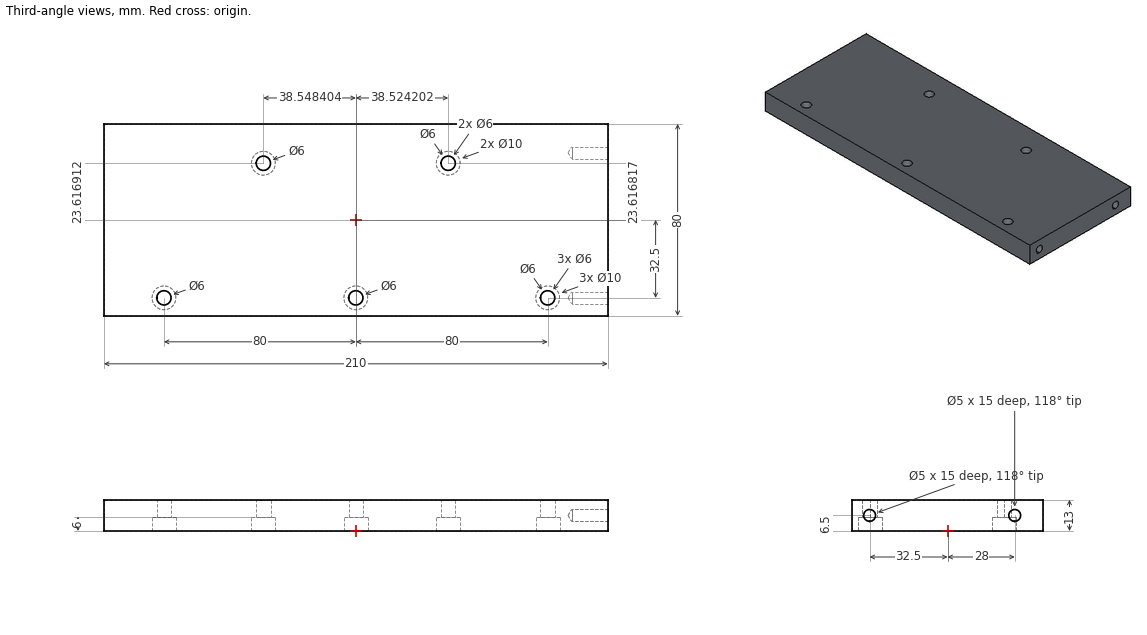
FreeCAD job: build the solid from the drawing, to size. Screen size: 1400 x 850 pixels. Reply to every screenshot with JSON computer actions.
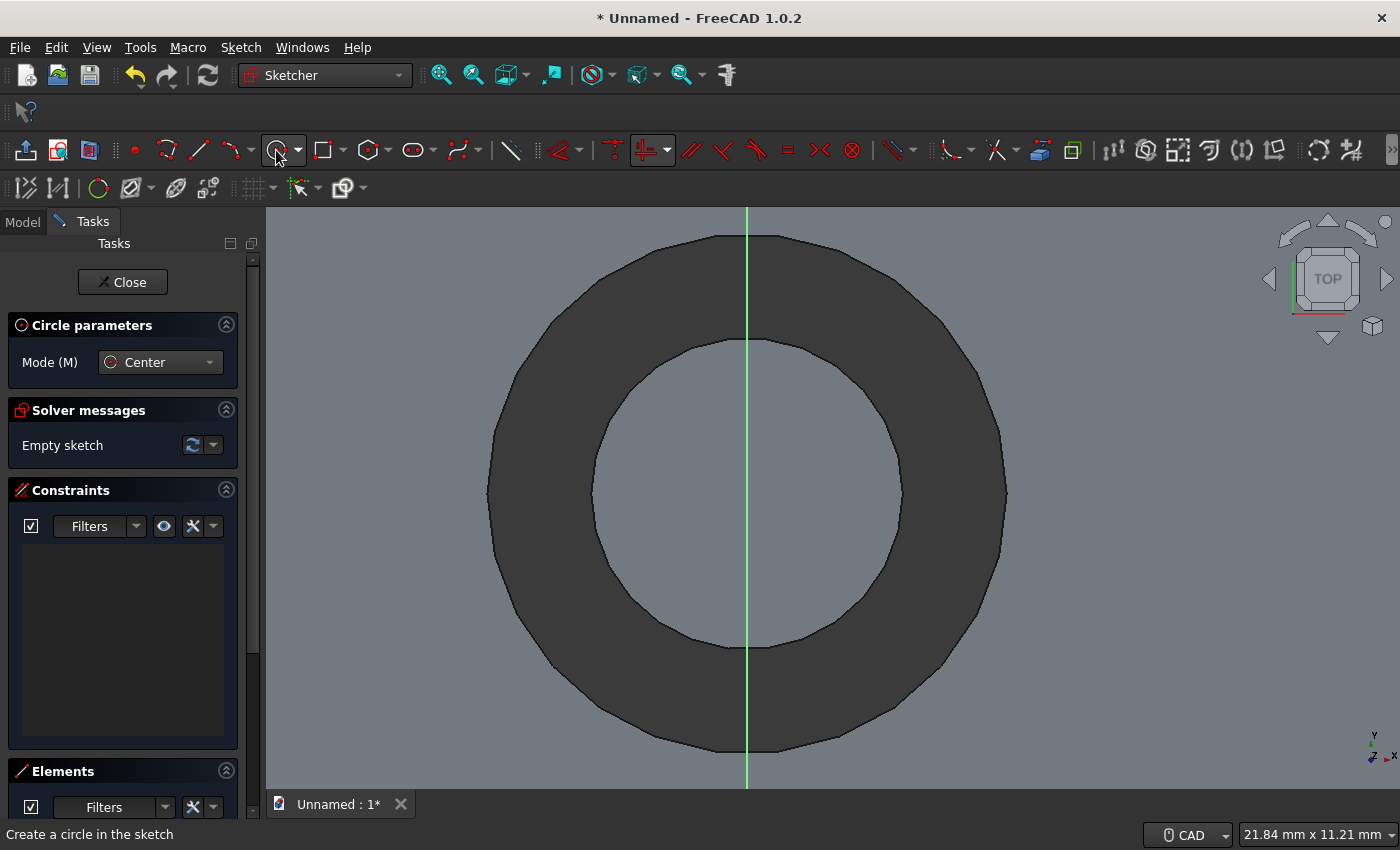
{"action": "left_click", "coordinate": [747, 494]}
{"action": "left_click", "coordinate": [857, 384]}
{"action": "key", "text": "Escape"}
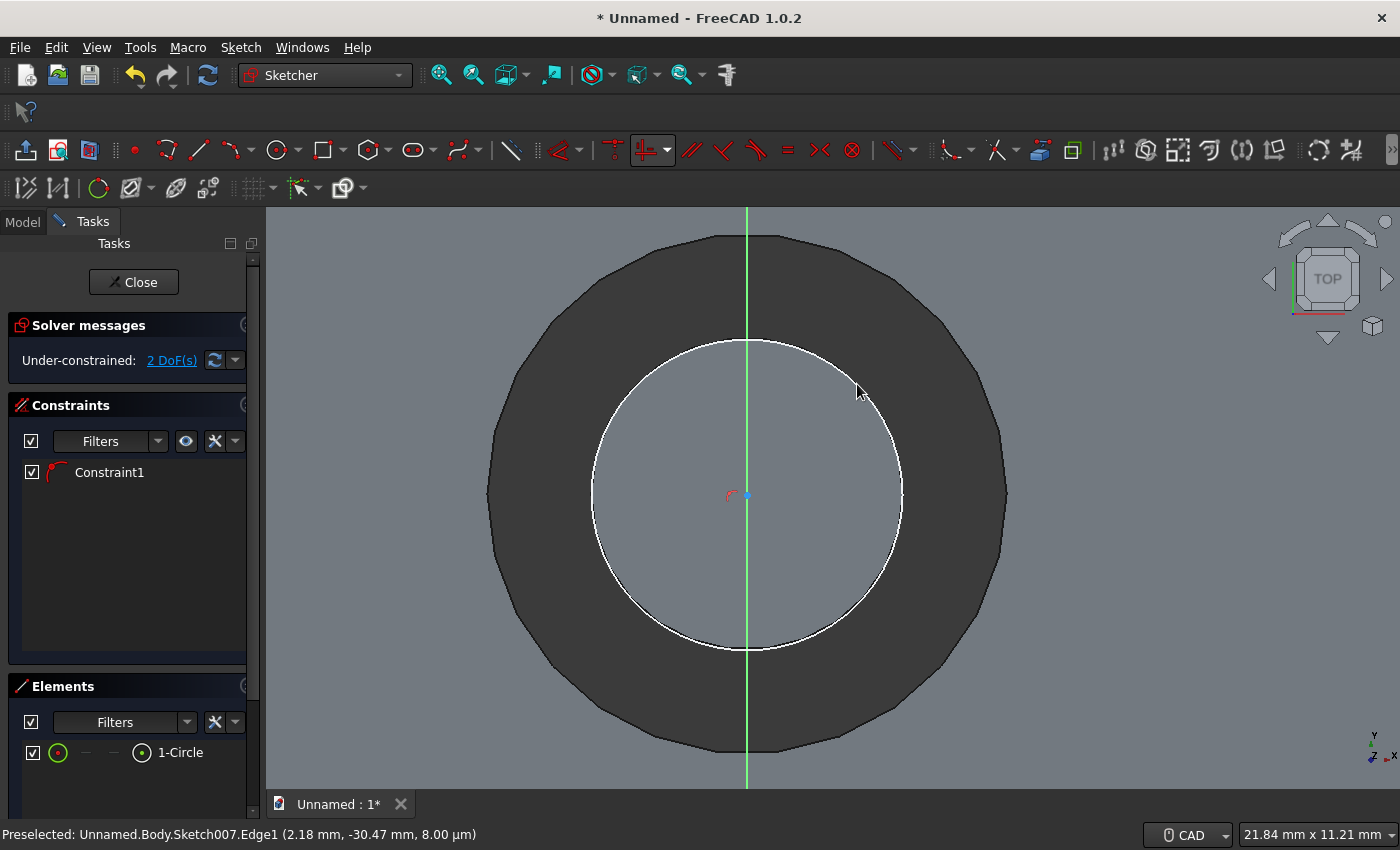
{"action": "key", "text": "d"}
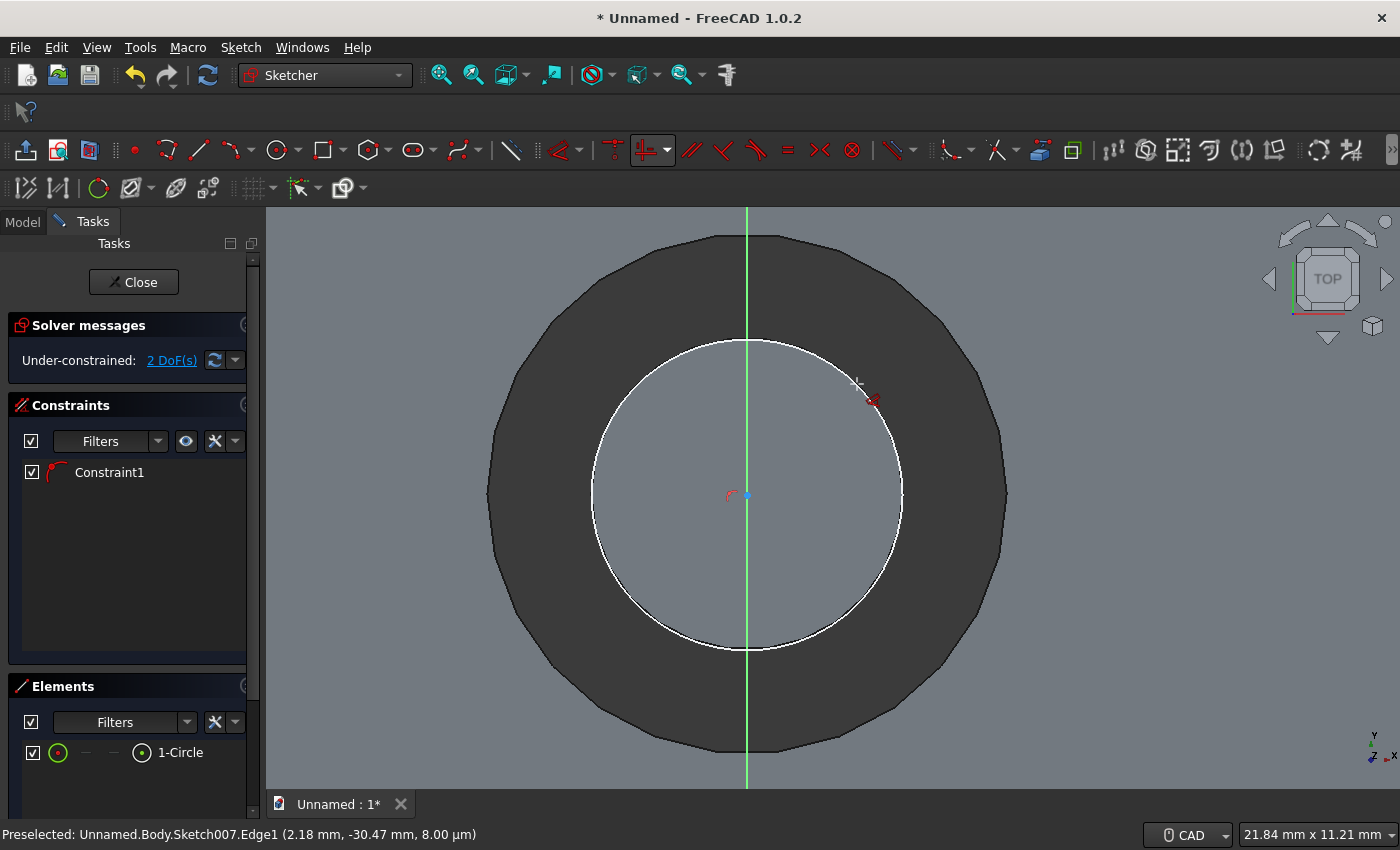
{"action": "left_click", "coordinate": [857, 385]}
{"action": "left_click", "coordinate": [880, 362]}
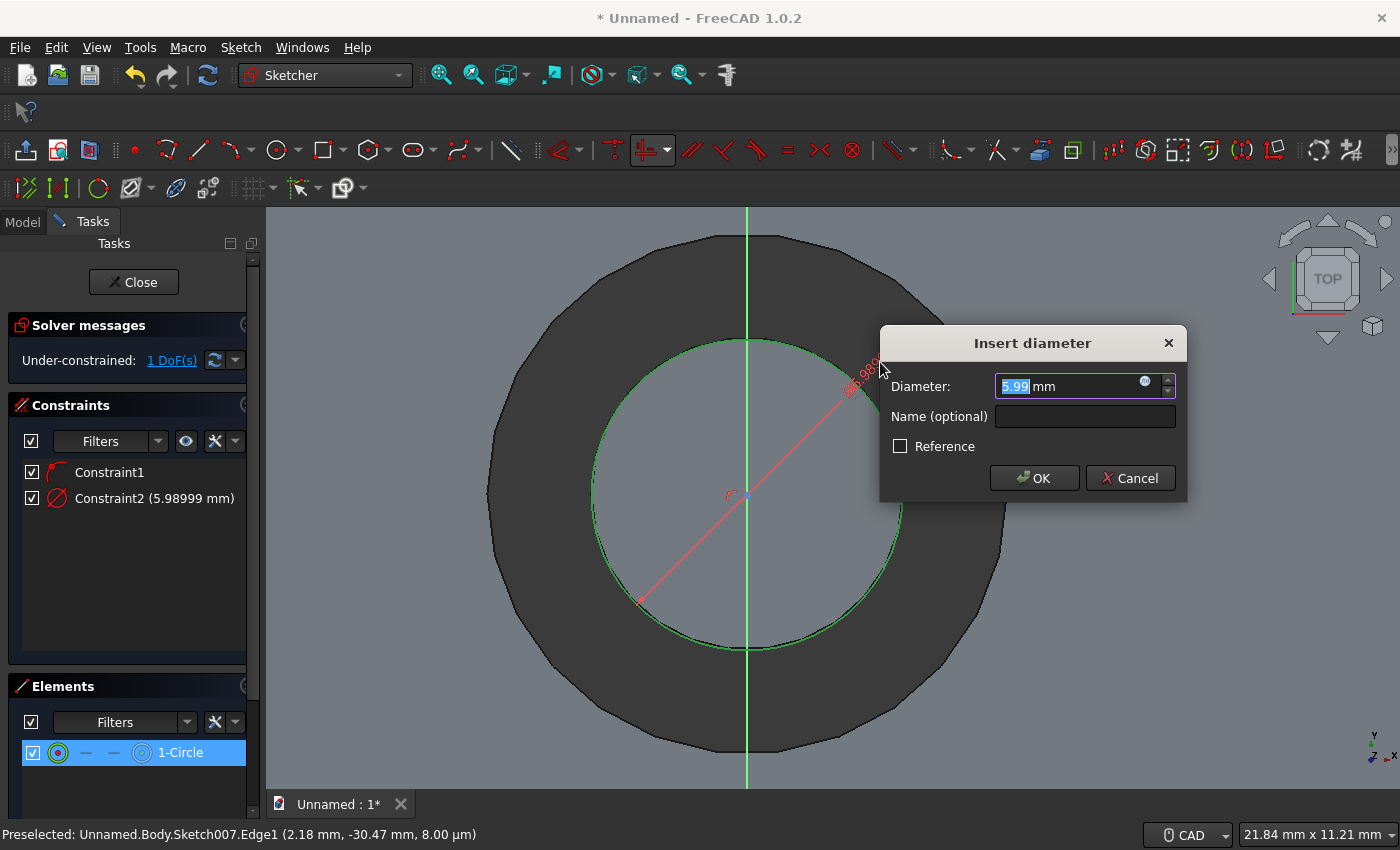
{"action": "type", "text": "6"}
{"action": "key", "text": "Return"}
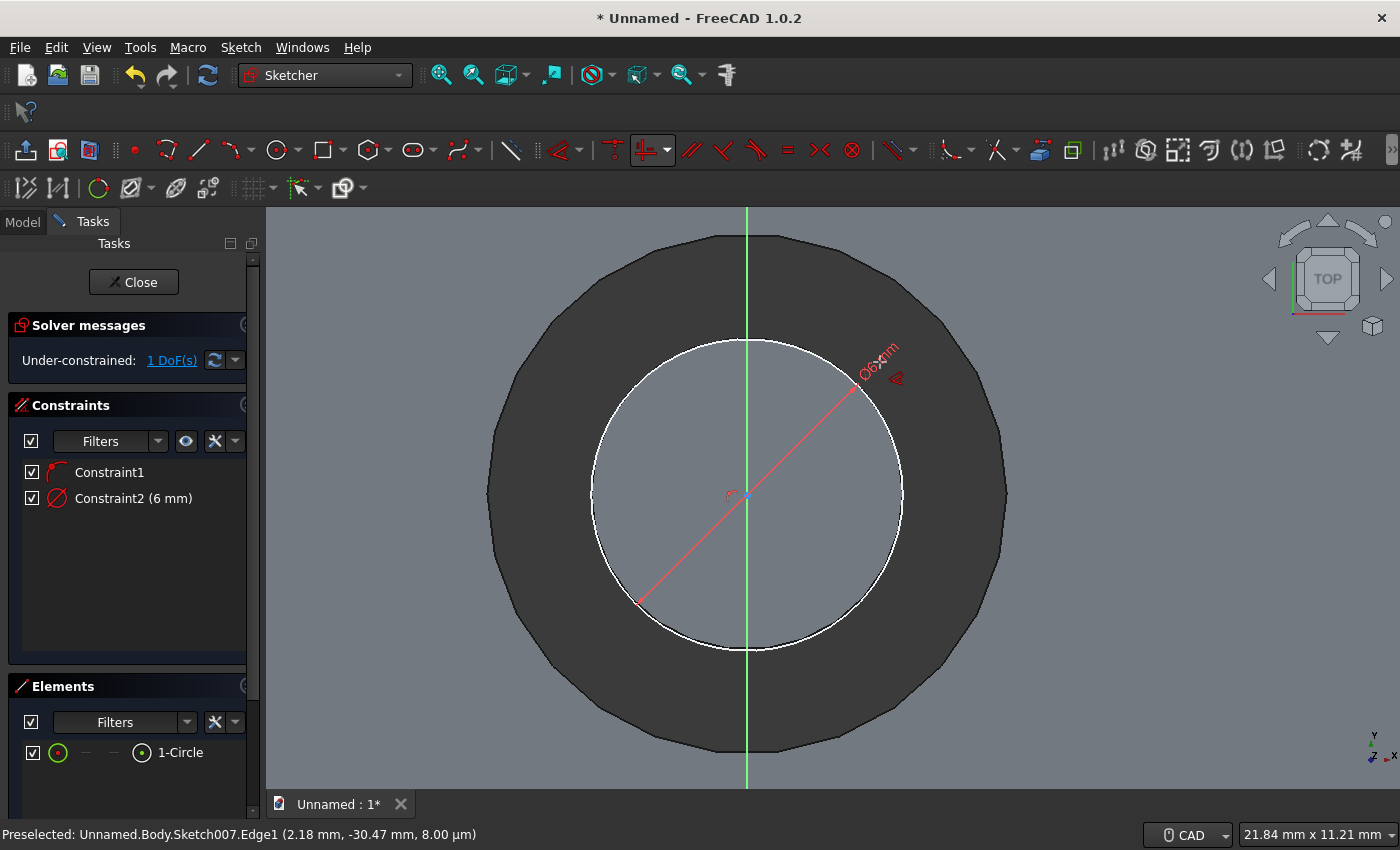
{"action": "left_click", "coordinate": [747, 495]}
{"action": "left_click", "coordinate": [781, 365]}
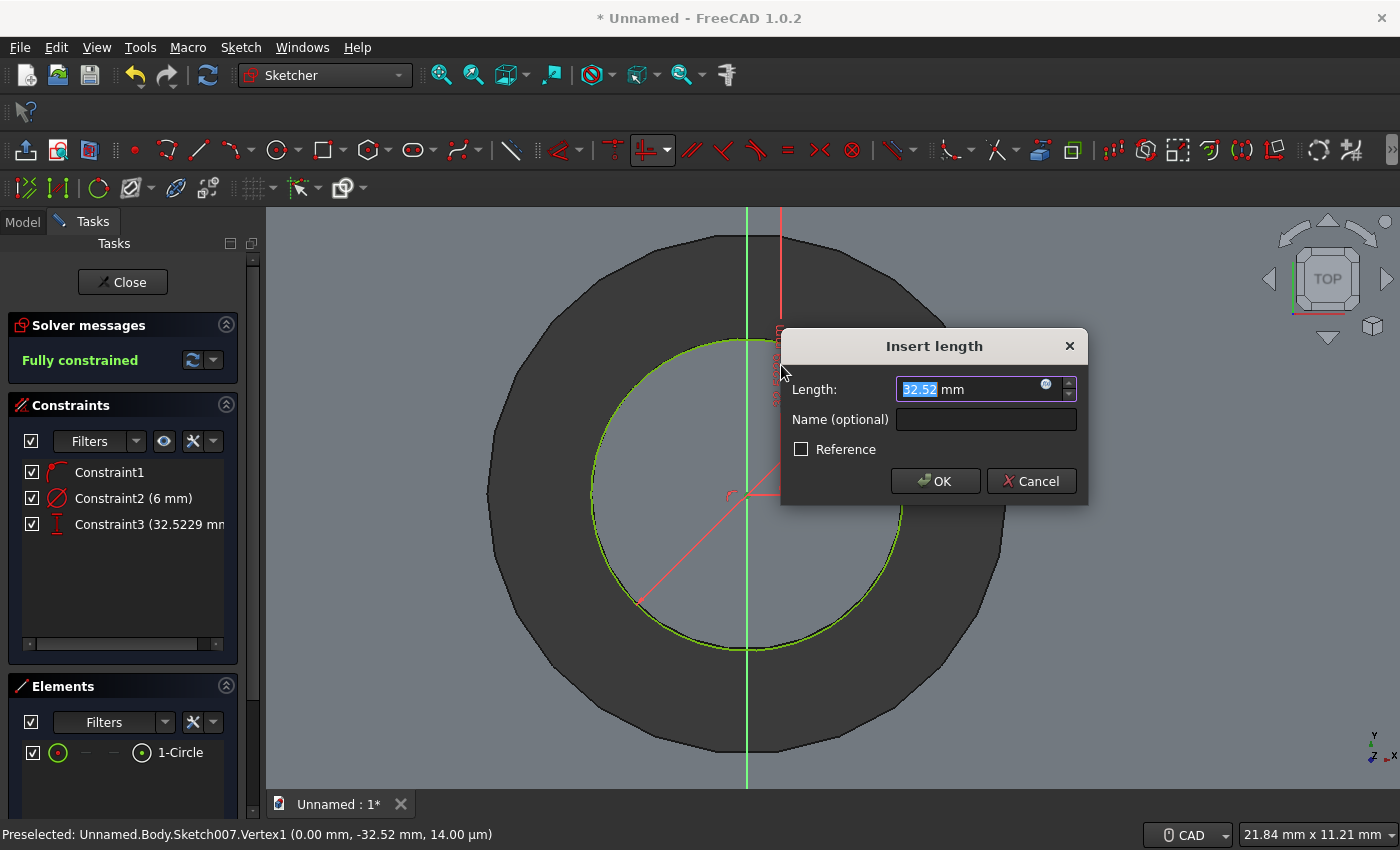
{"action": "type", "text": "32.5"}
{"action": "key", "text": "Return"}
{"action": "key", "text": "Escape"}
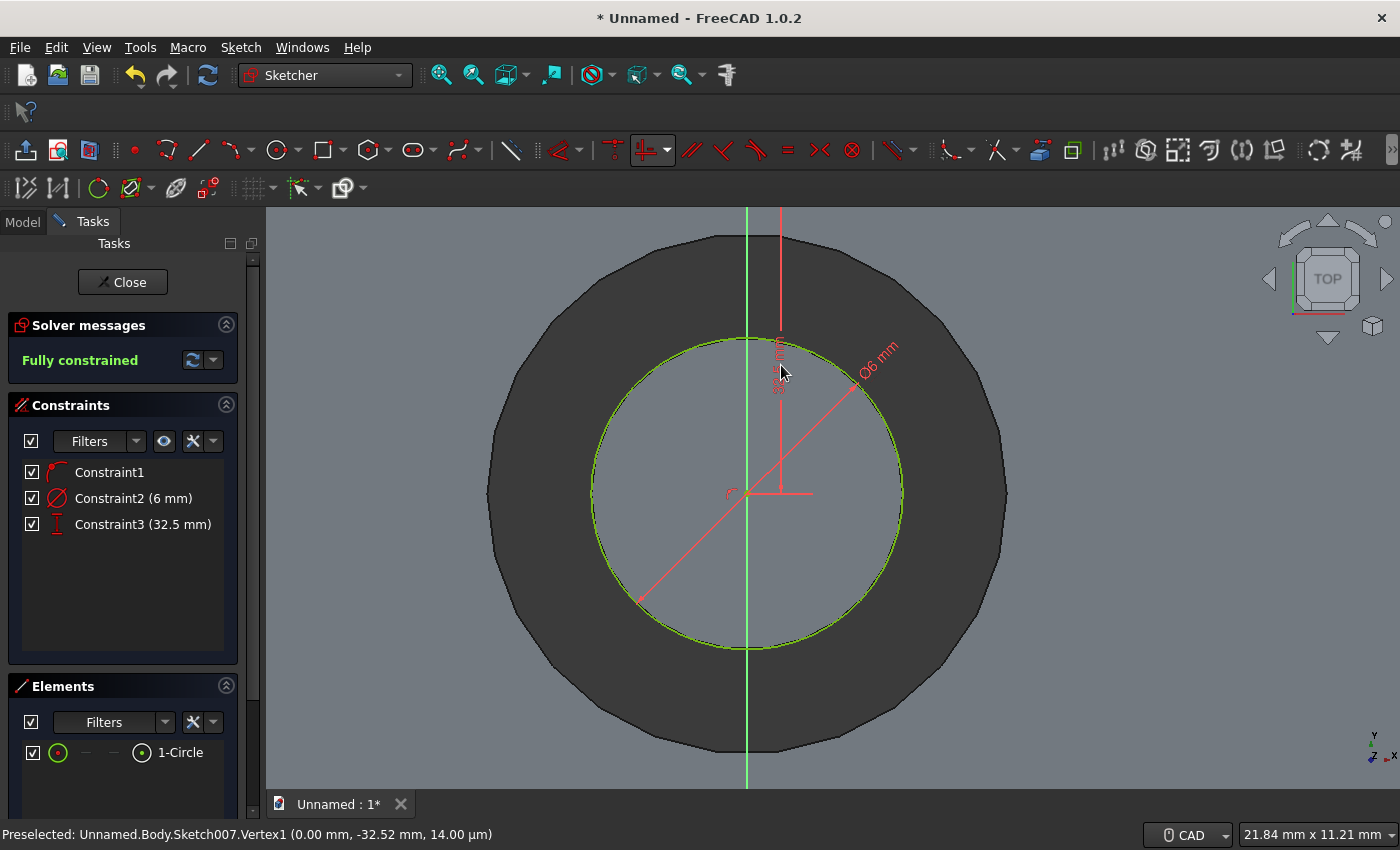
{"action": "left_click", "coordinate": [123, 282]}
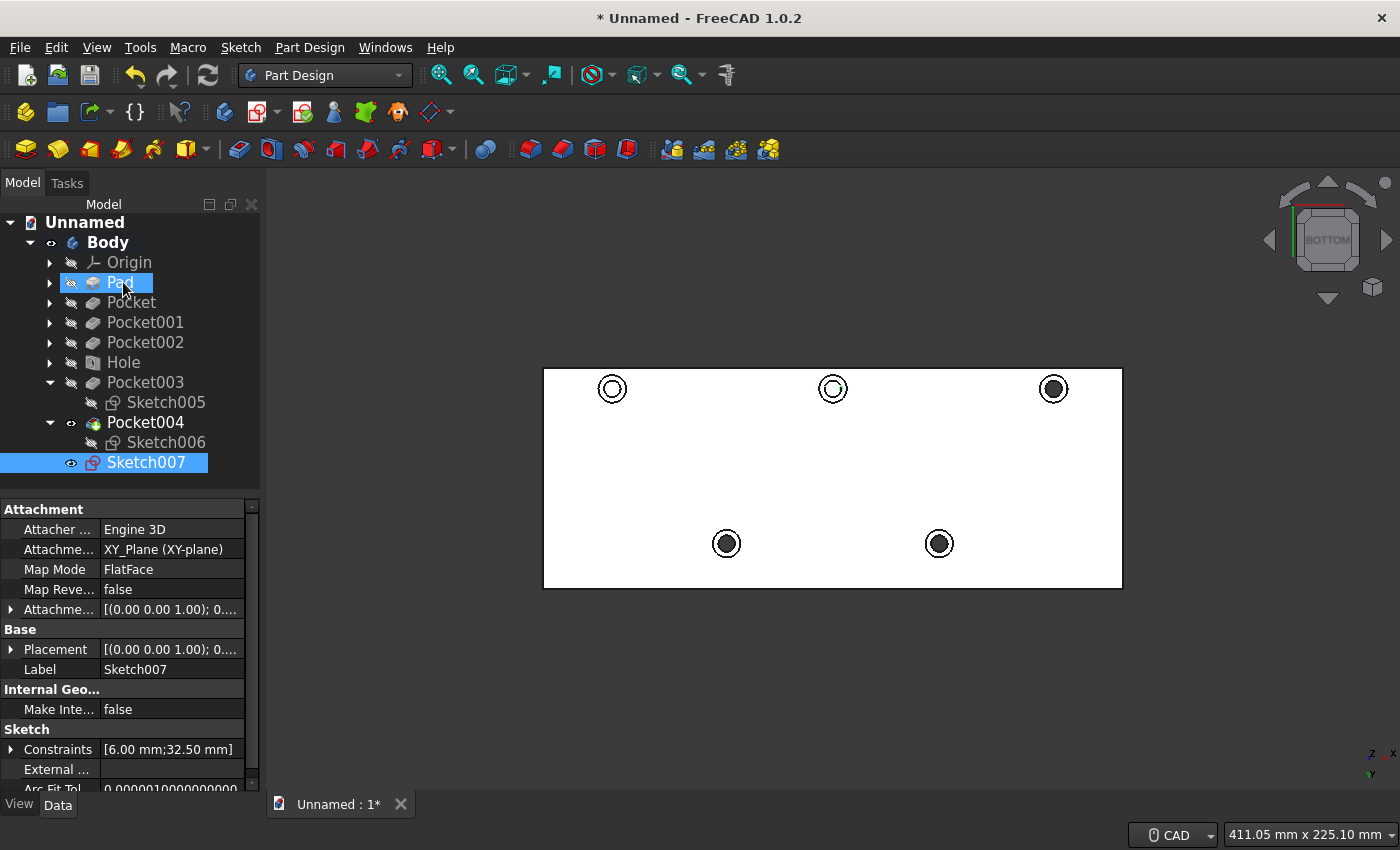
{"action": "left_click", "coordinate": [240, 150]}